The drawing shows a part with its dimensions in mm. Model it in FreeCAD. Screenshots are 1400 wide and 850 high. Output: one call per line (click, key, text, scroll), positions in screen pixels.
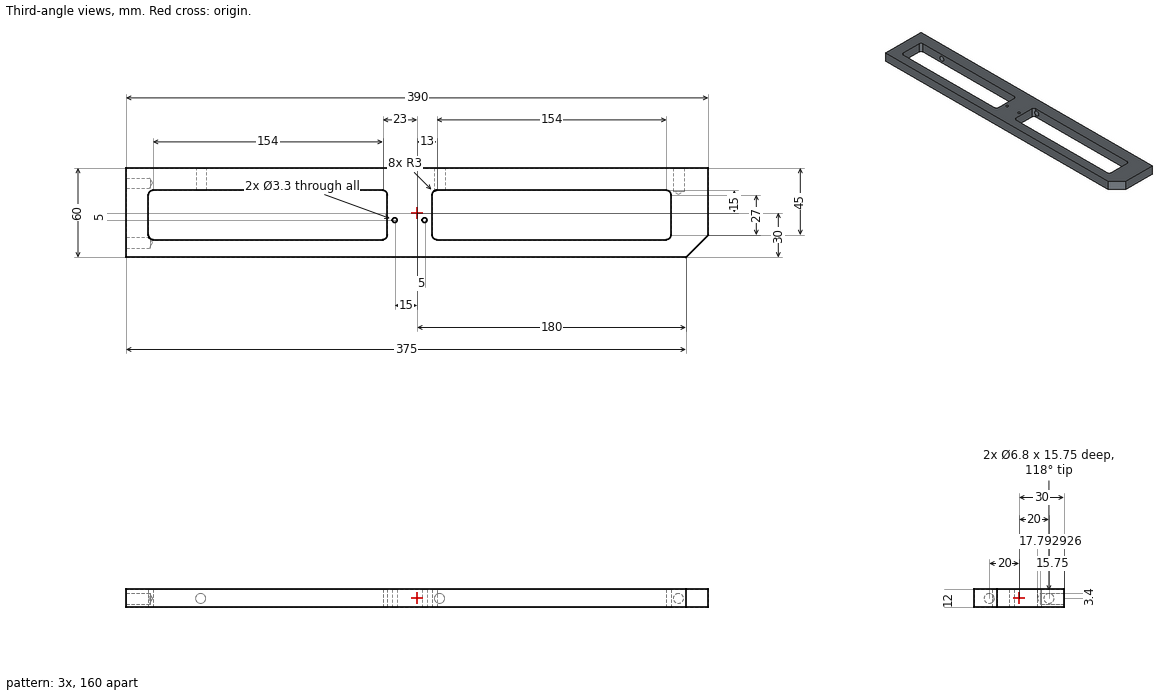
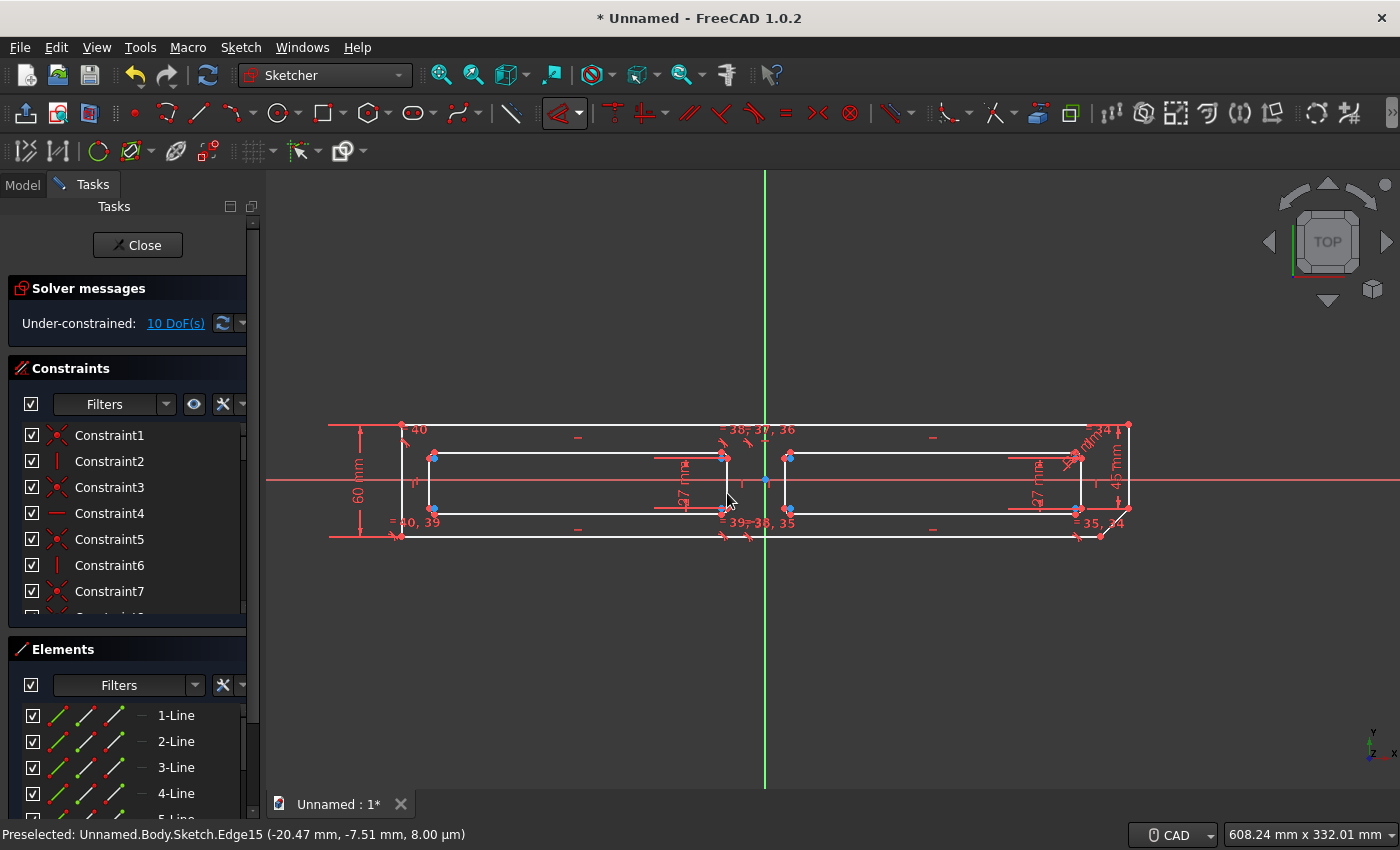
click(911, 425)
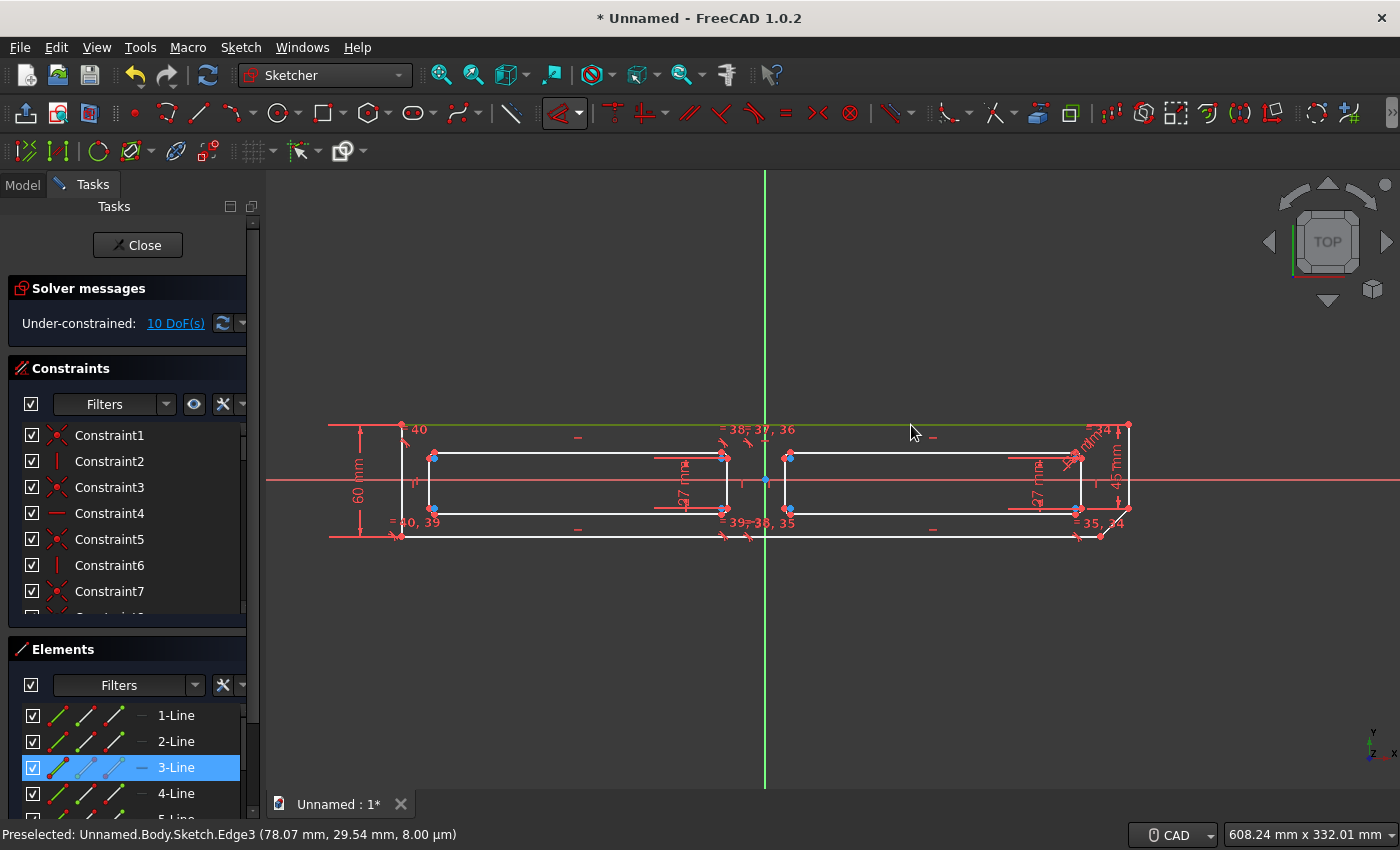
key(l)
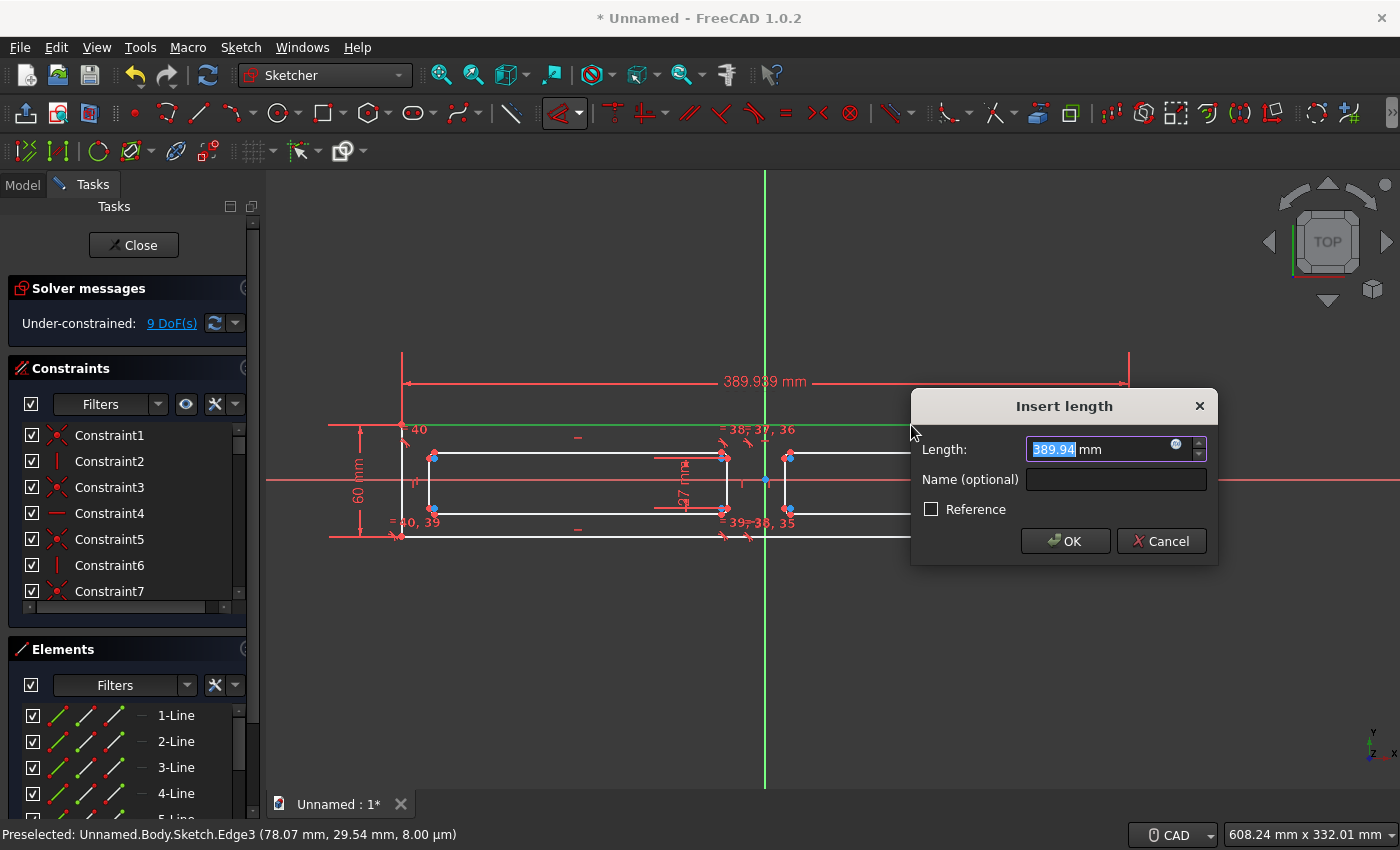
text(390)
key(Return)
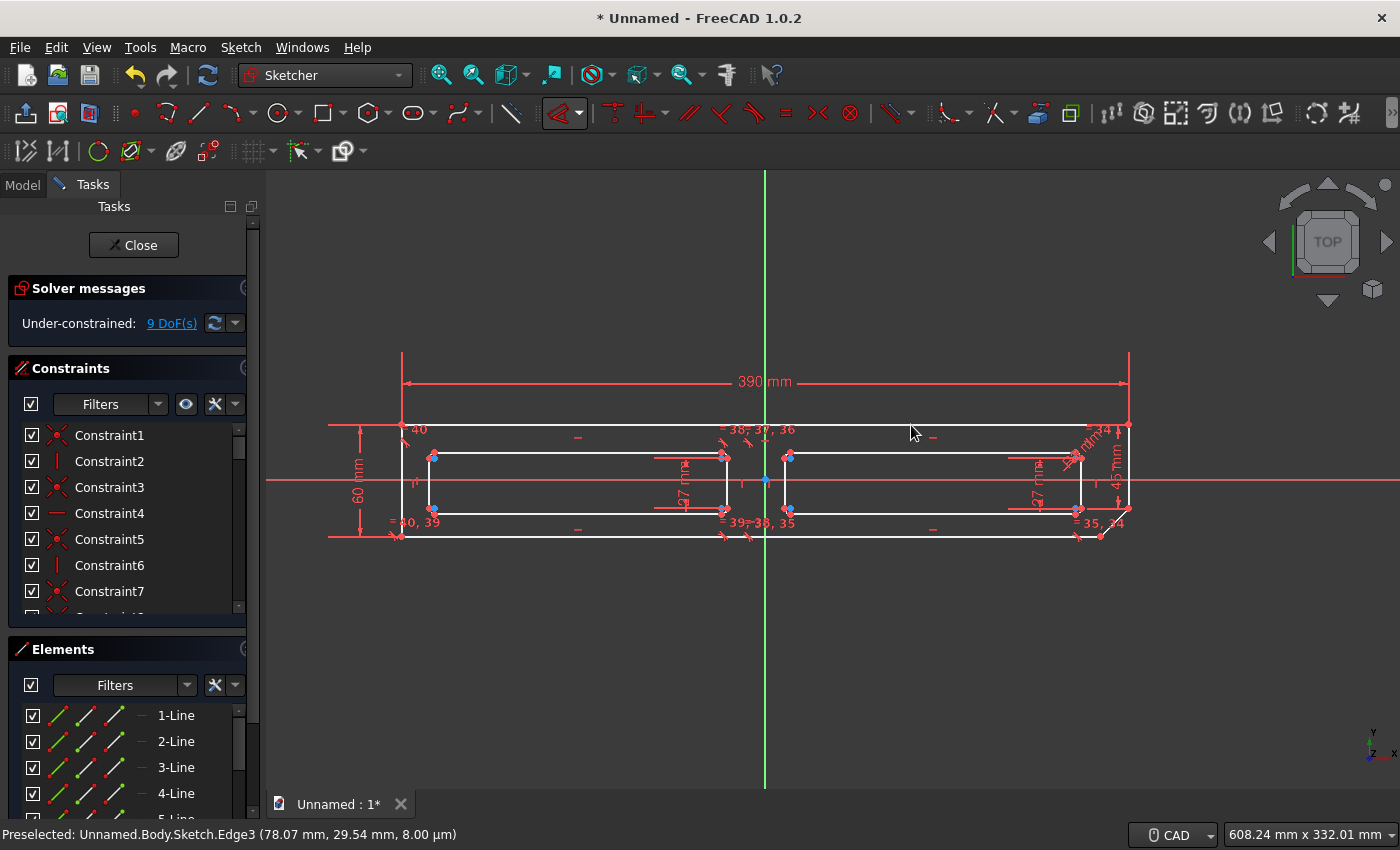
click(611, 537)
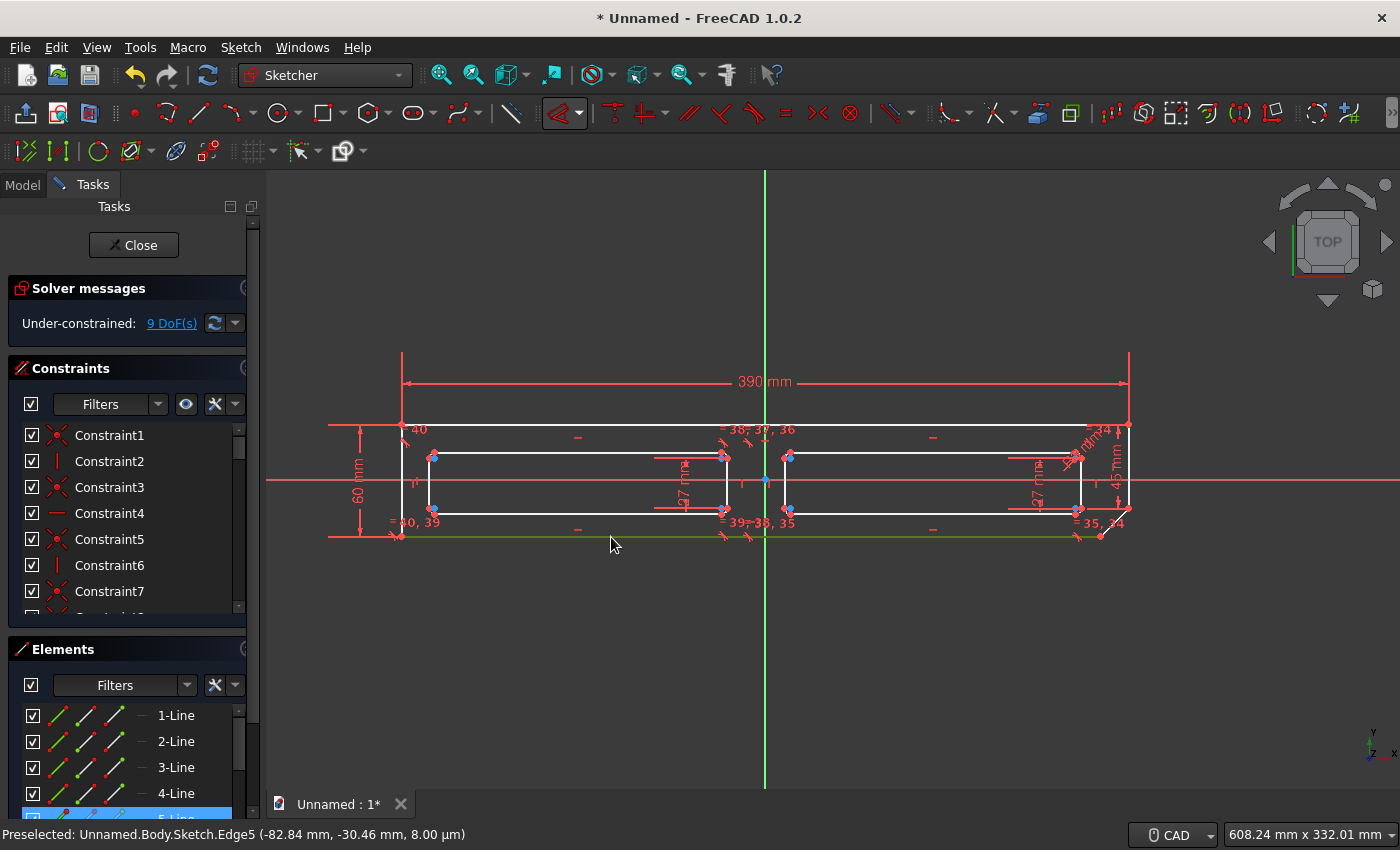
click(582, 114)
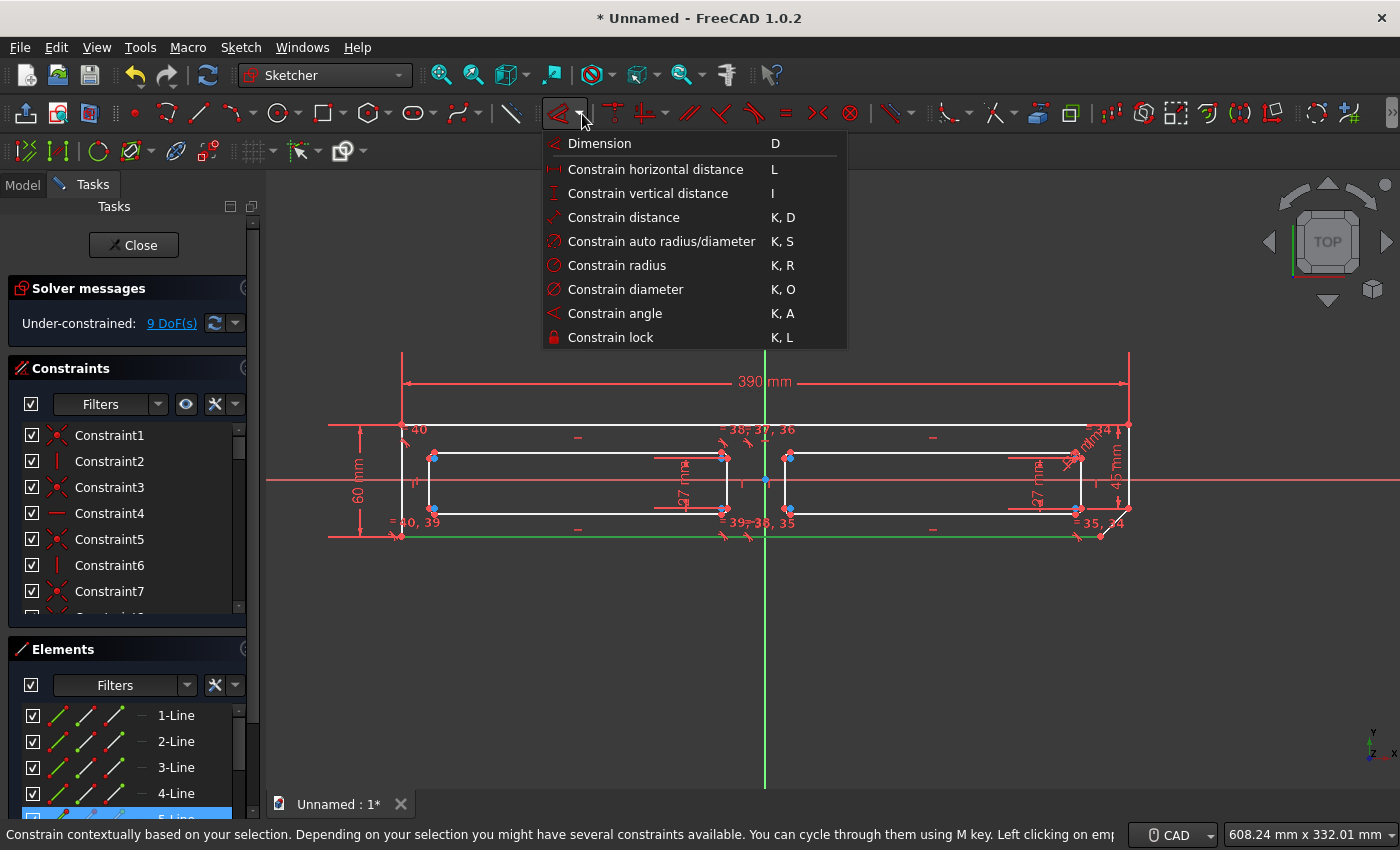
click(695, 169)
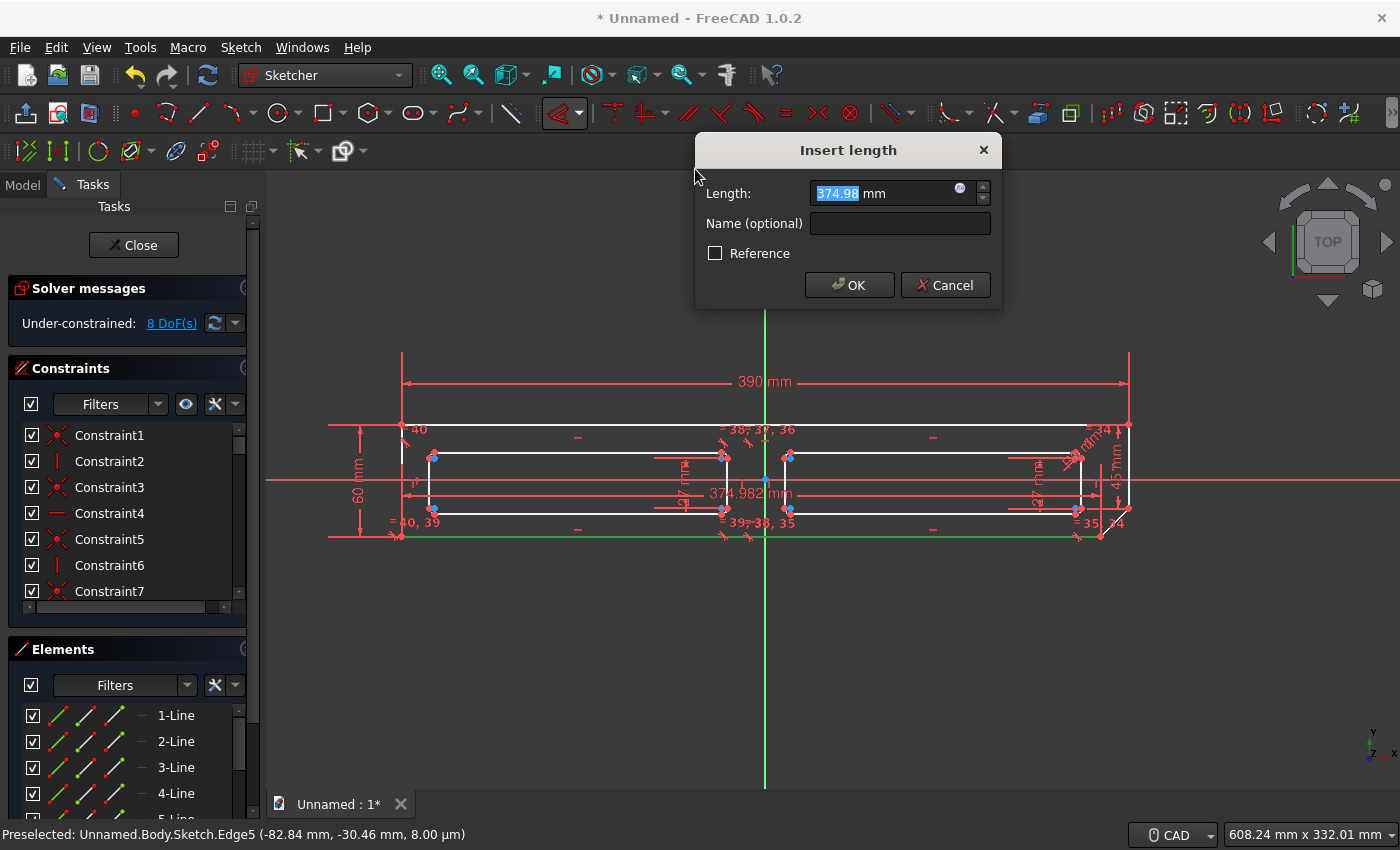
text(375)
key(Return)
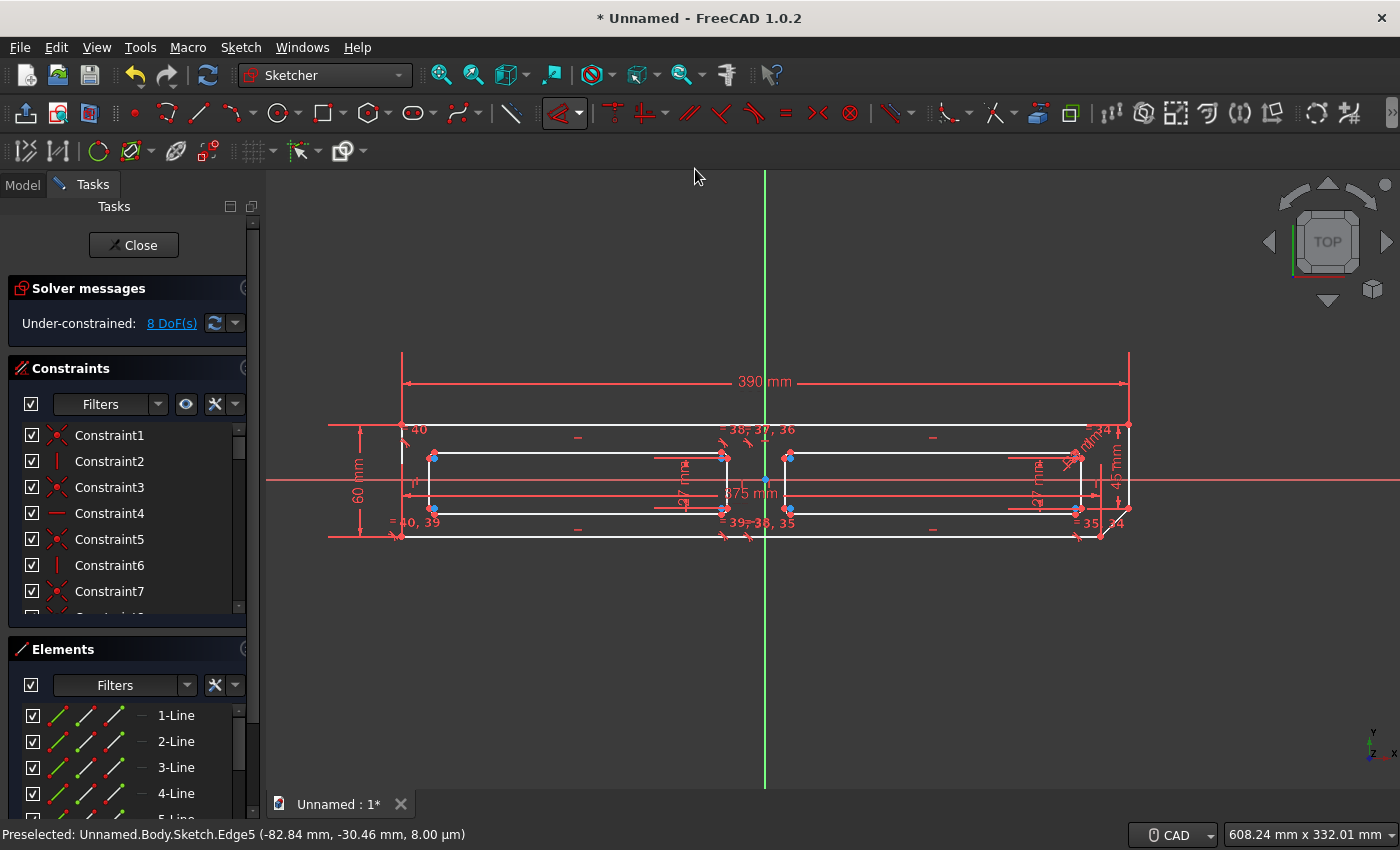
click(876, 453)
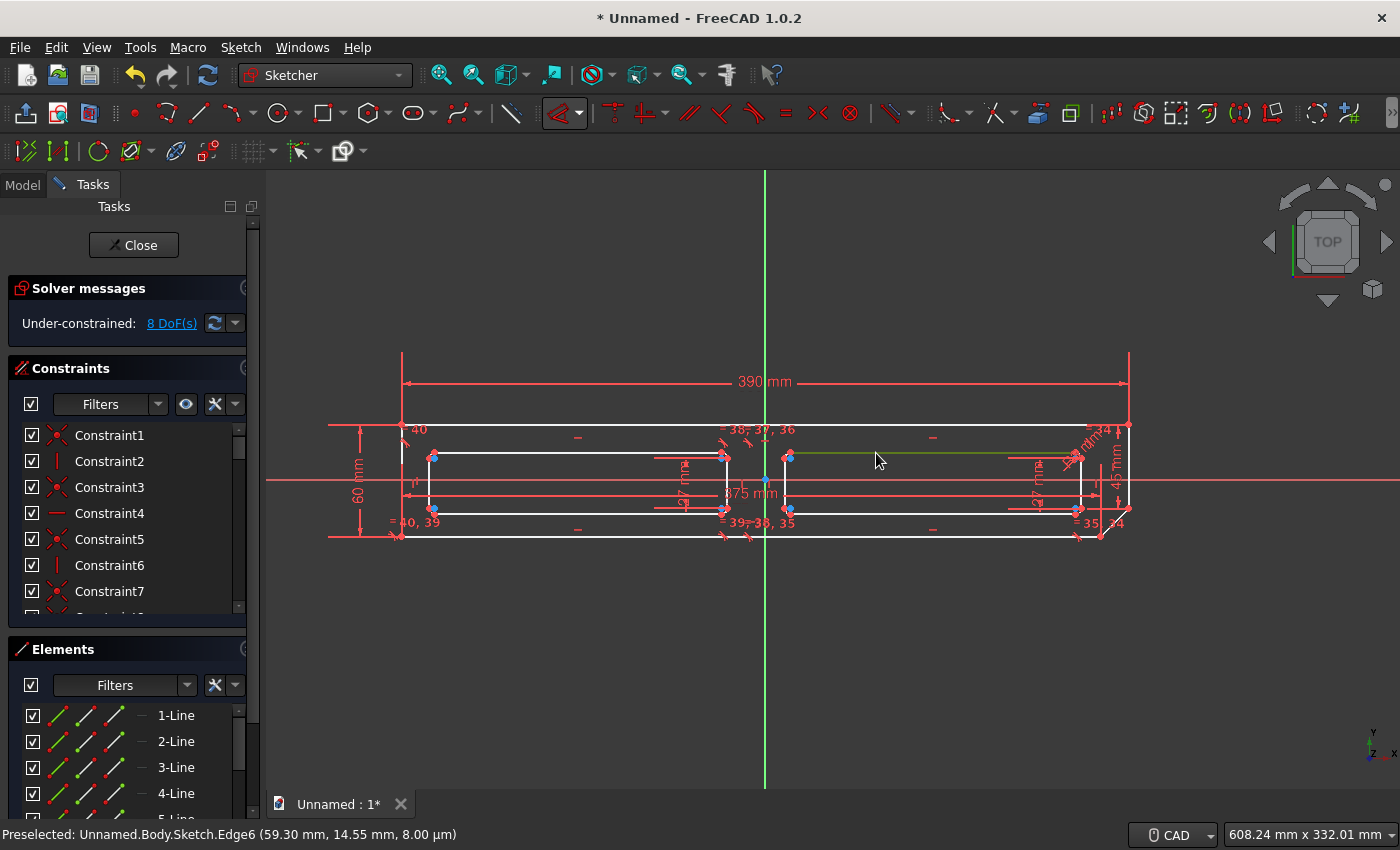
click(582, 114)